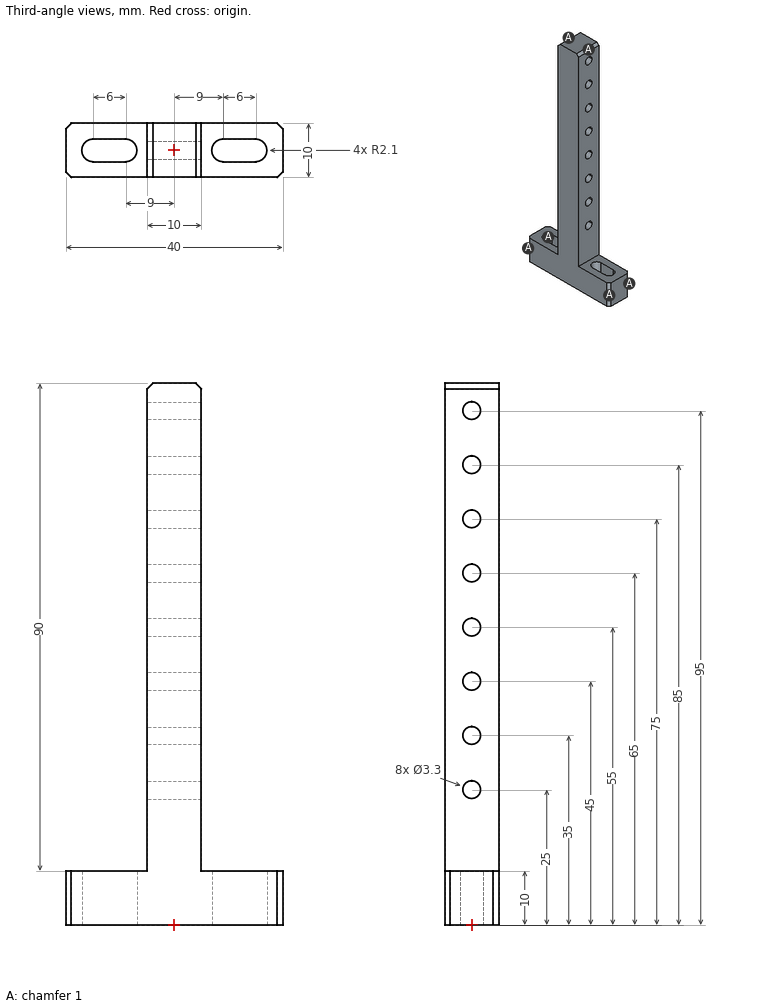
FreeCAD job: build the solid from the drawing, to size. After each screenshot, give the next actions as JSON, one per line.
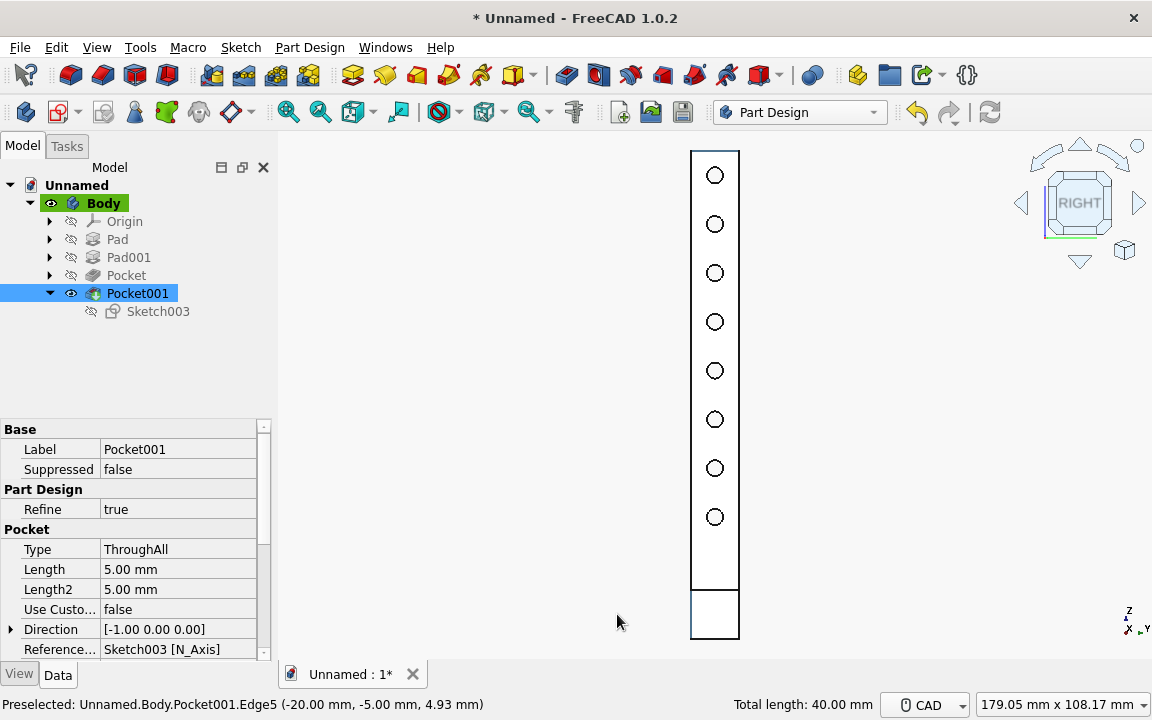
{"action": "left_click", "coordinate": [739, 614], "text": "ctrl"}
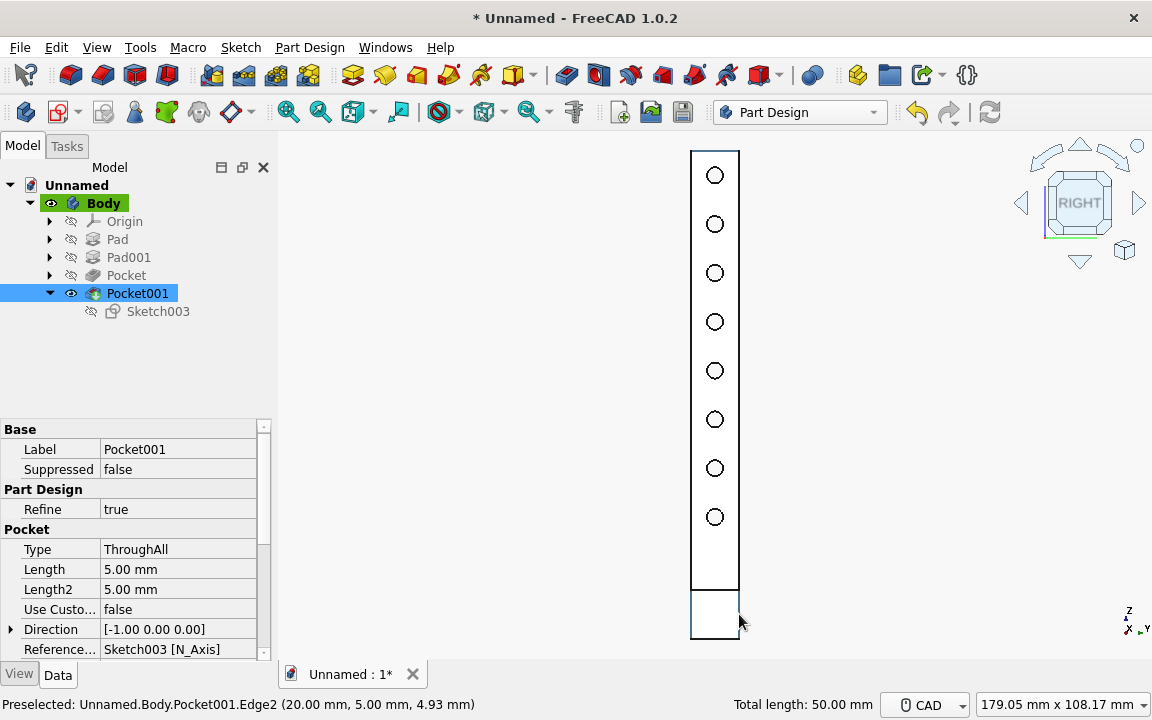
{"action": "key", "text": "5"}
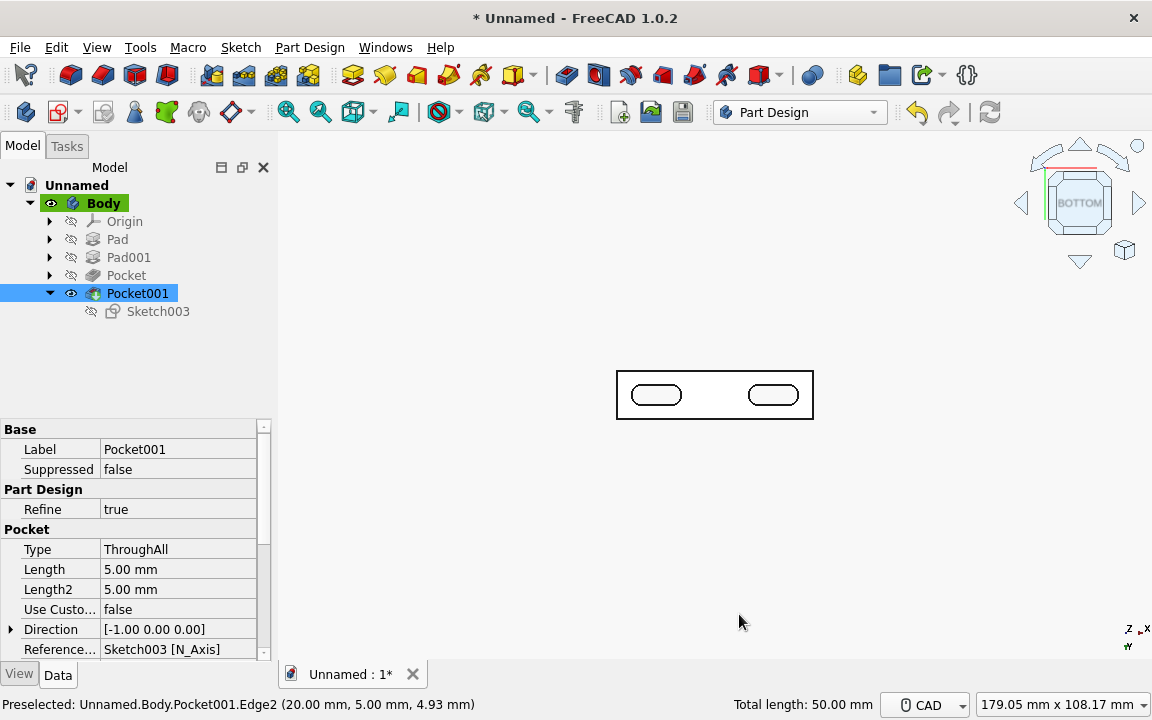
{"action": "left_click", "coordinate": [290, 112]}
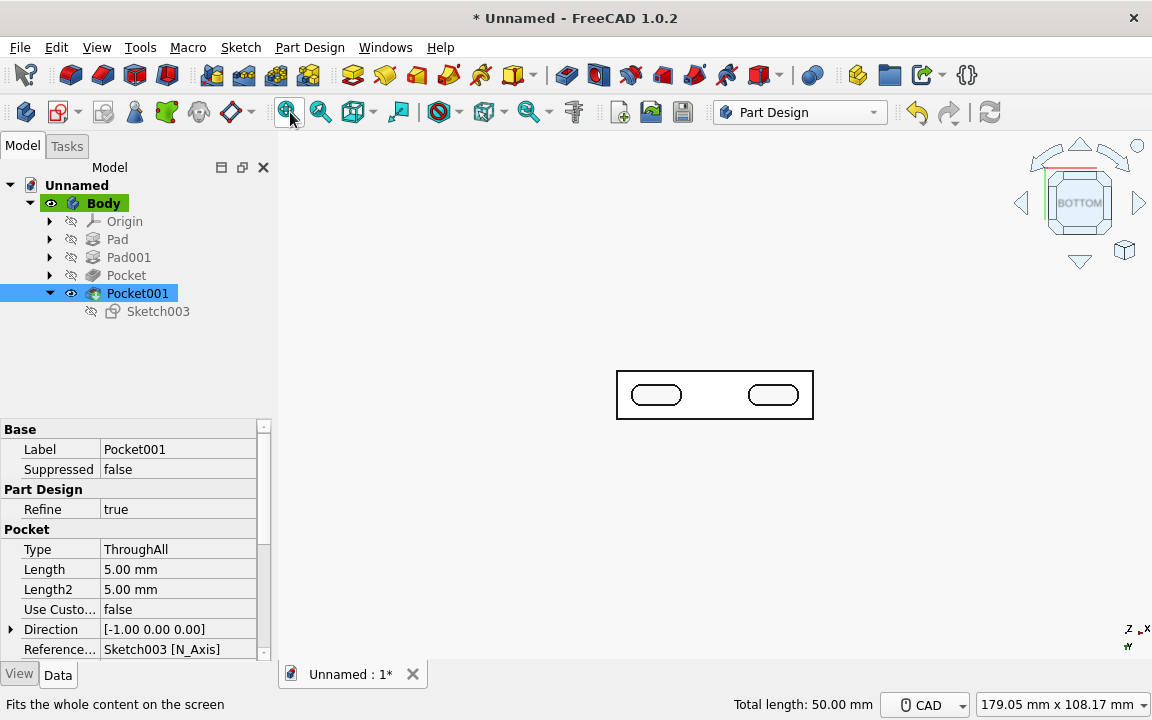
{"action": "key", "text": "4"}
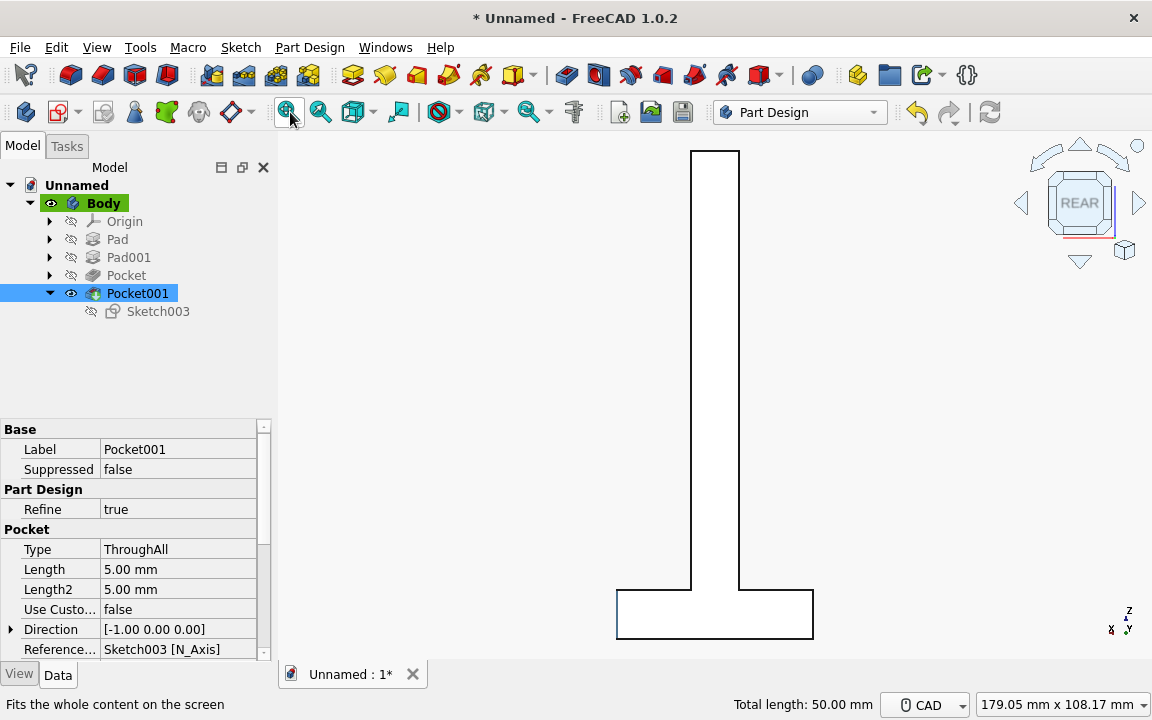
{"action": "left_click", "coordinate": [813, 614], "text": "ctrl"}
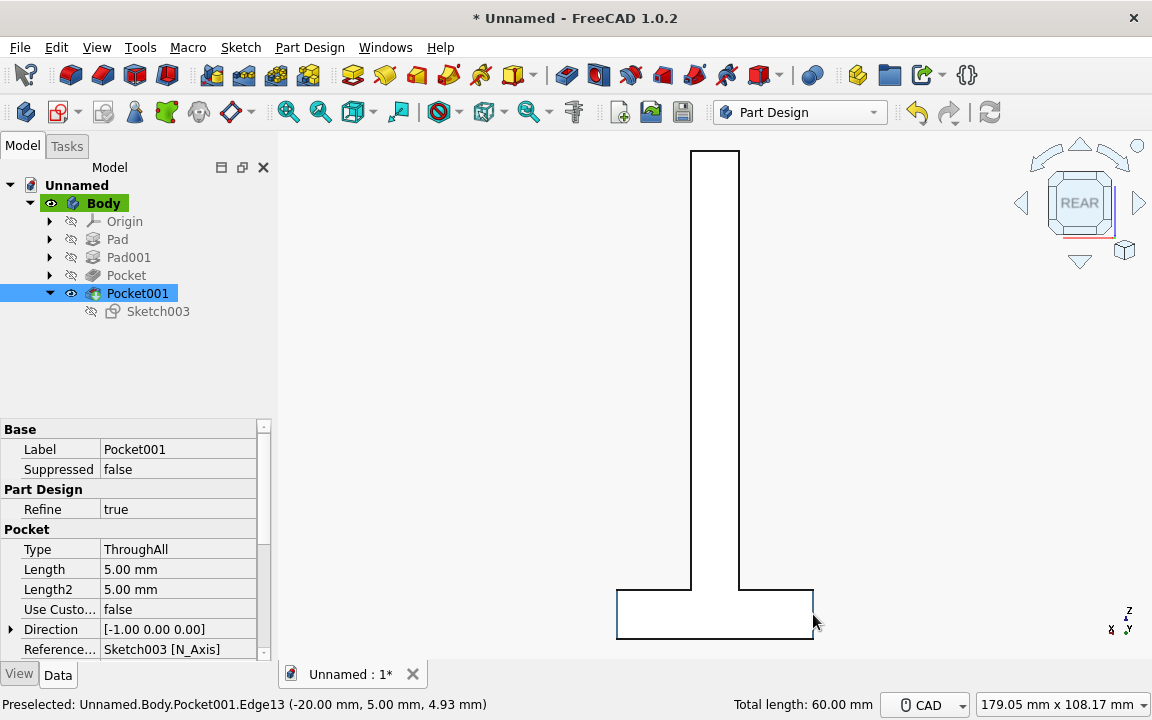
{"action": "left_click", "coordinate": [104, 76]}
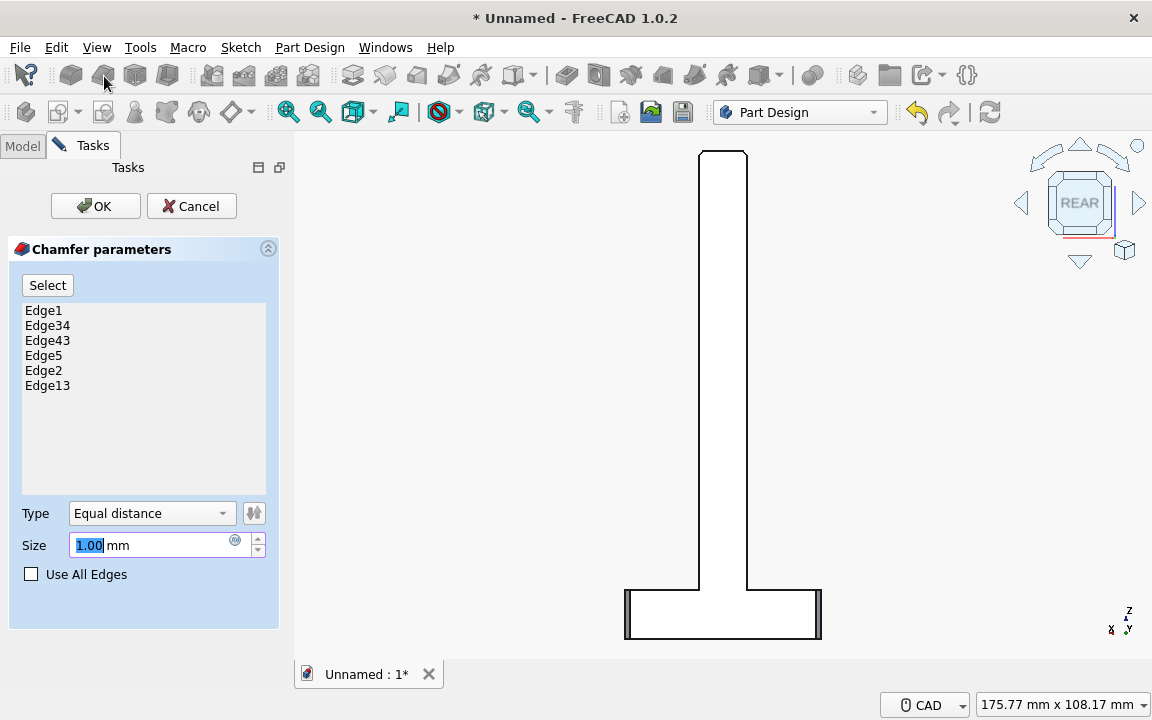
{"action": "type", "text": "1"}
{"action": "key", "text": "Tab"}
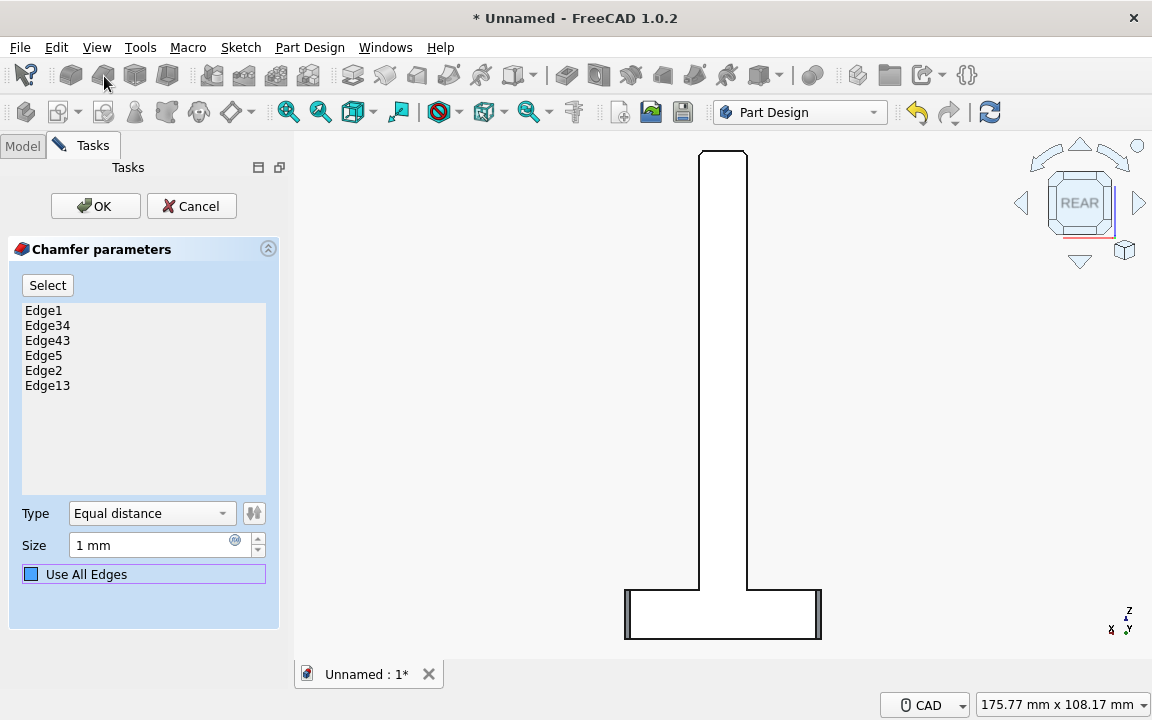
{"action": "left_click", "coordinate": [96, 206]}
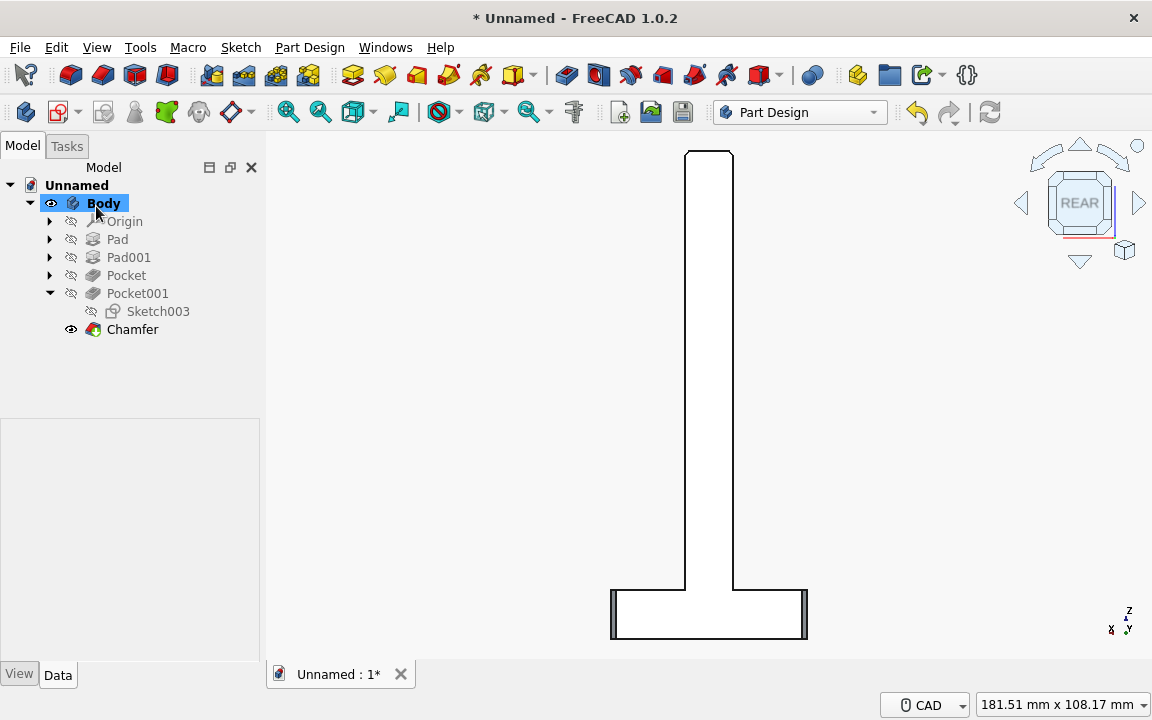
{"action": "key", "text": "0"}